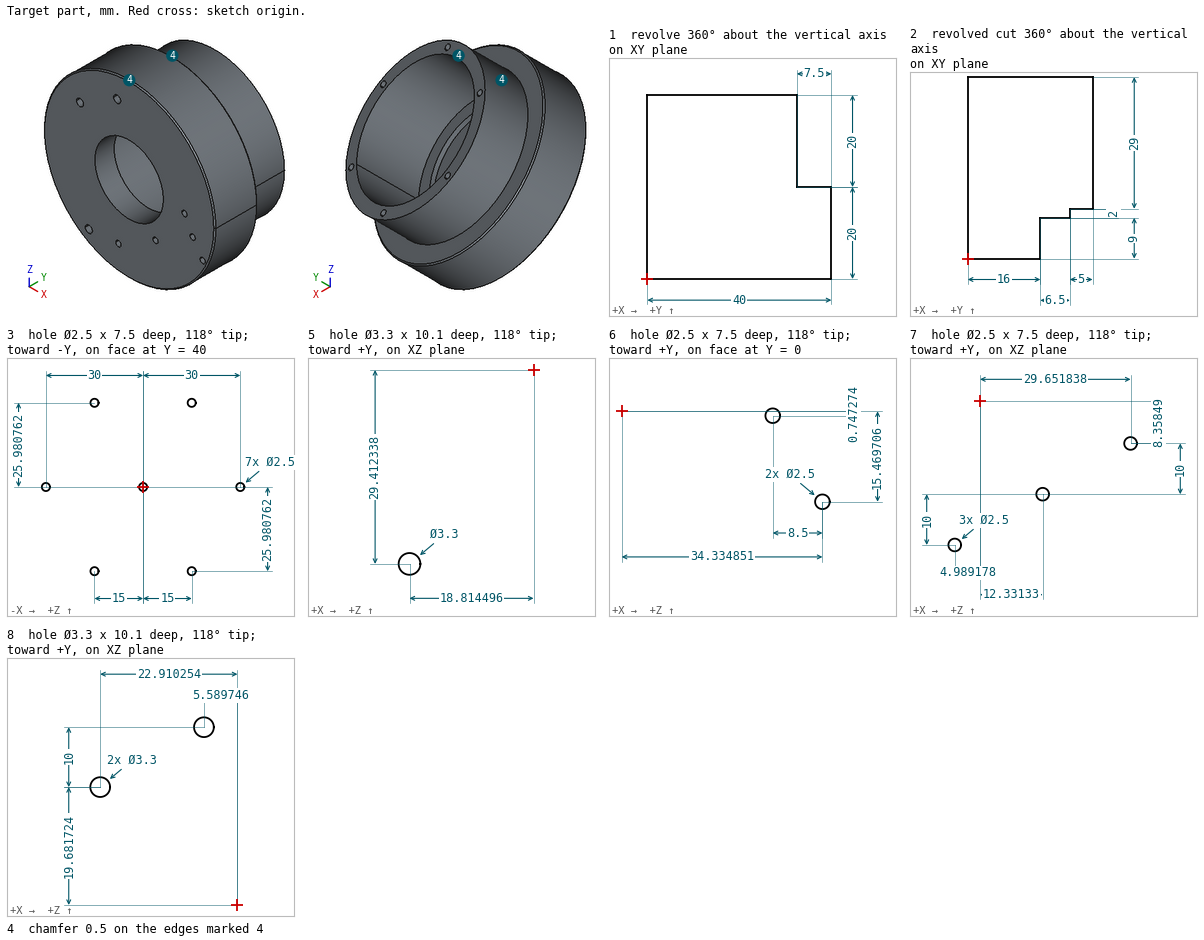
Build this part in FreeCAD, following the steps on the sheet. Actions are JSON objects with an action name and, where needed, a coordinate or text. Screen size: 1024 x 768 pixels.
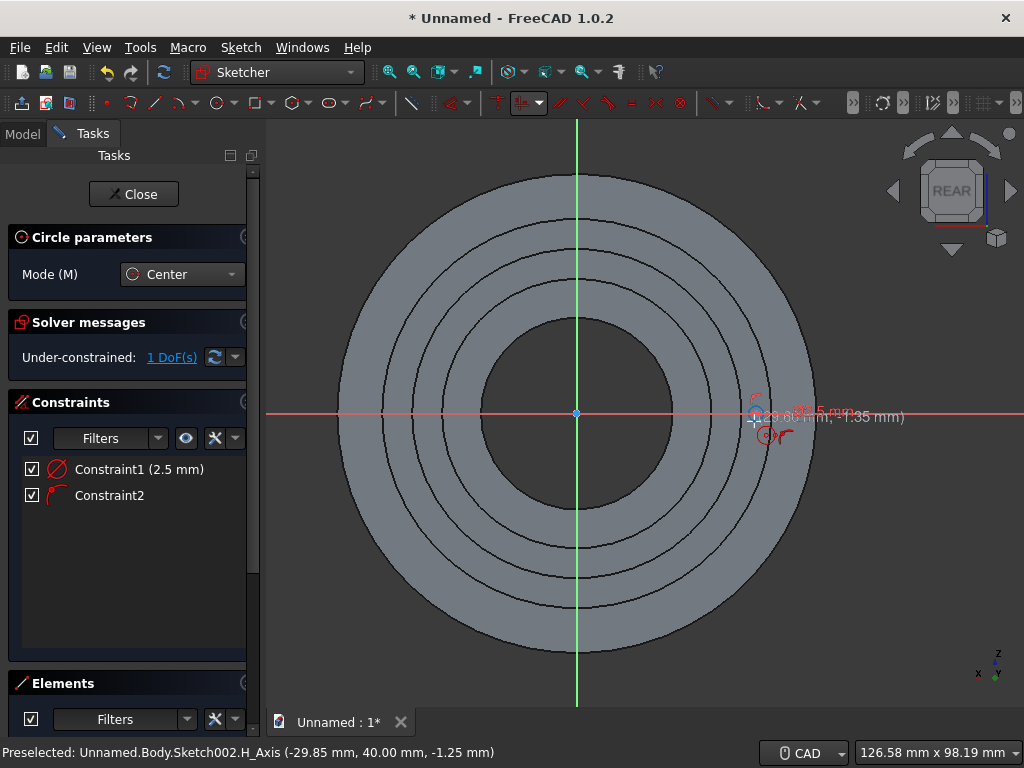
{"action": "scroll", "coordinate": [667, 569], "scroll_direction": "up", "scroll_amount": 6}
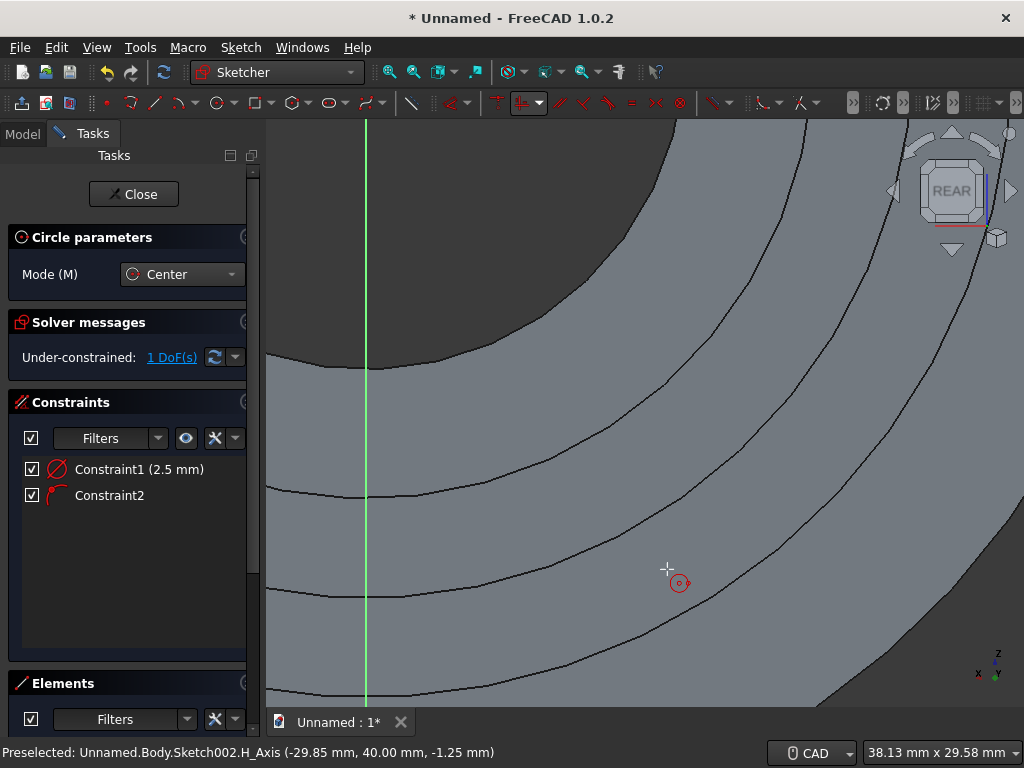
{"action": "scroll", "coordinate": [667, 569], "scroll_direction": "down", "scroll_amount": 6}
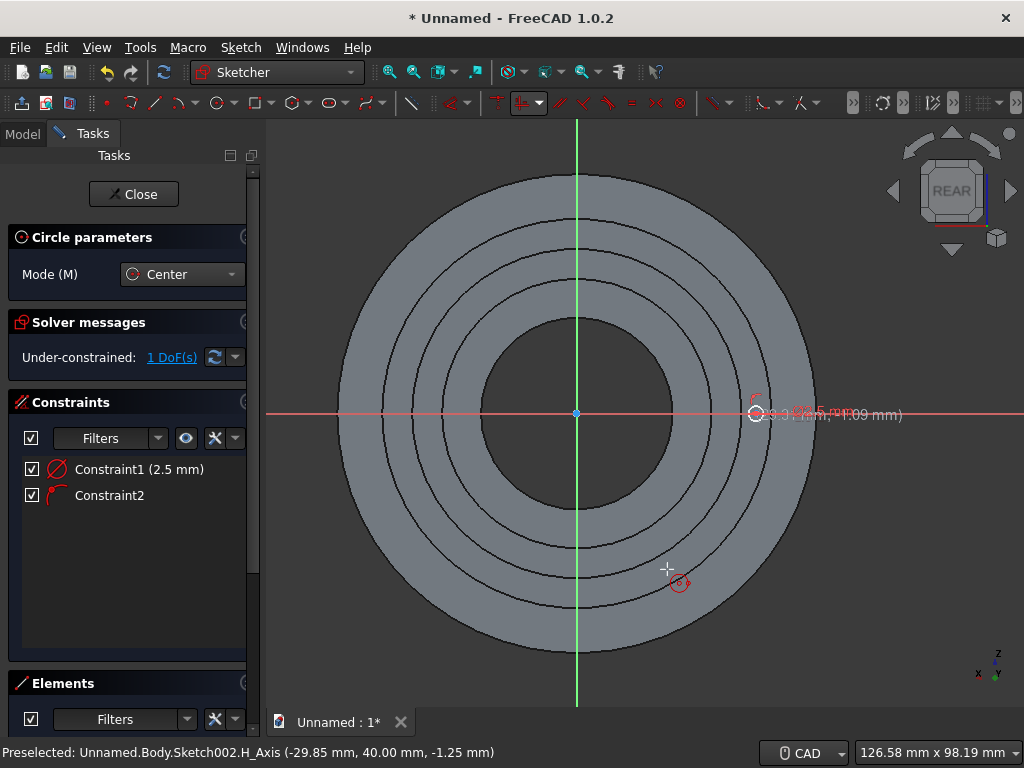
{"action": "left_click", "coordinate": [667, 569]}
{"action": "mouse_move", "coordinate": [672, 564]}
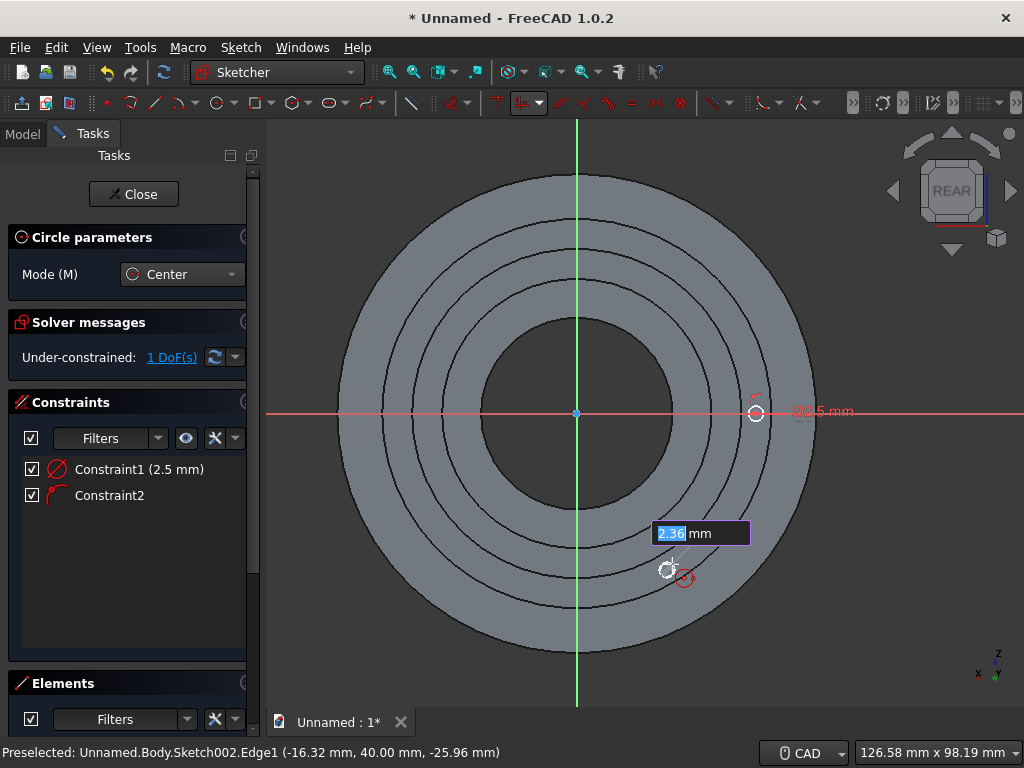
{"action": "type", "text": "2.5"}
{"action": "key", "text": "Return"}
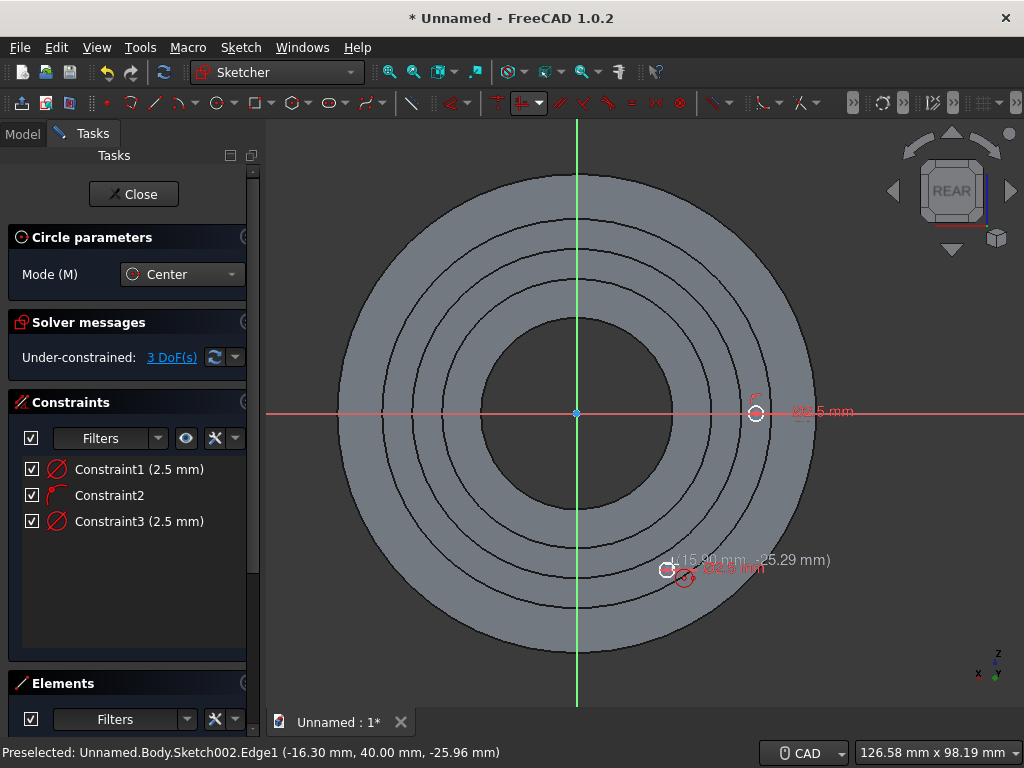
{"action": "scroll", "coordinate": [487, 569], "scroll_direction": "up", "scroll_amount": 6}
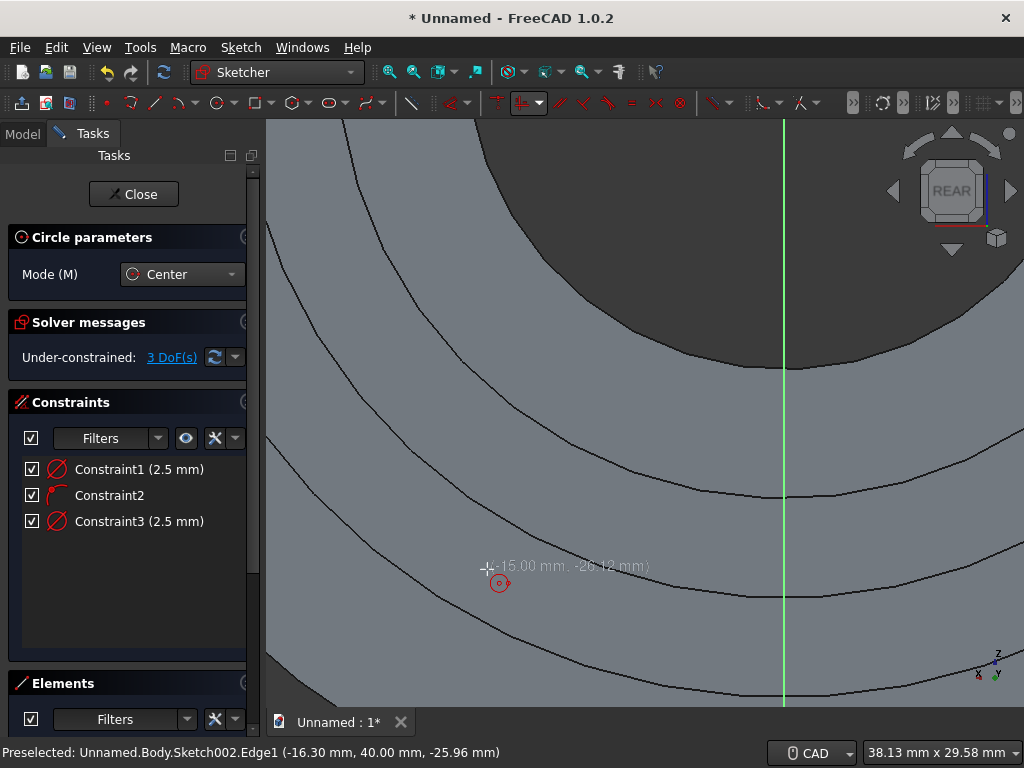
{"action": "scroll", "coordinate": [487, 569], "scroll_direction": "down", "scroll_amount": 6}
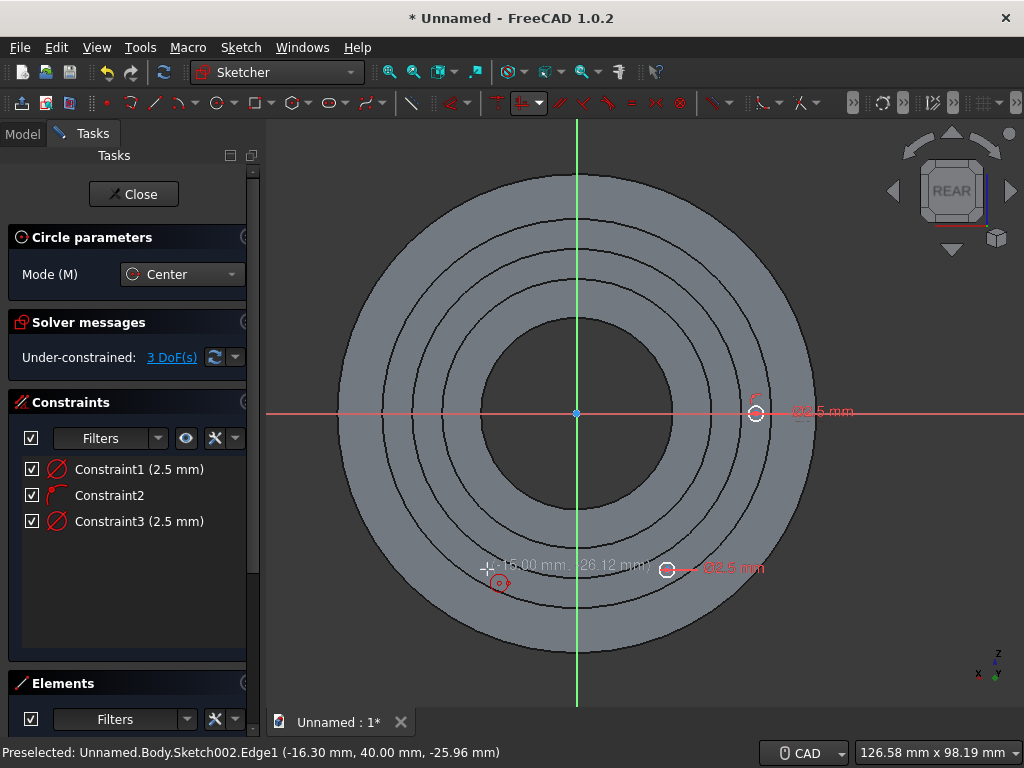
{"action": "left_click", "coordinate": [487, 569]}
{"action": "mouse_move", "coordinate": [492, 564]}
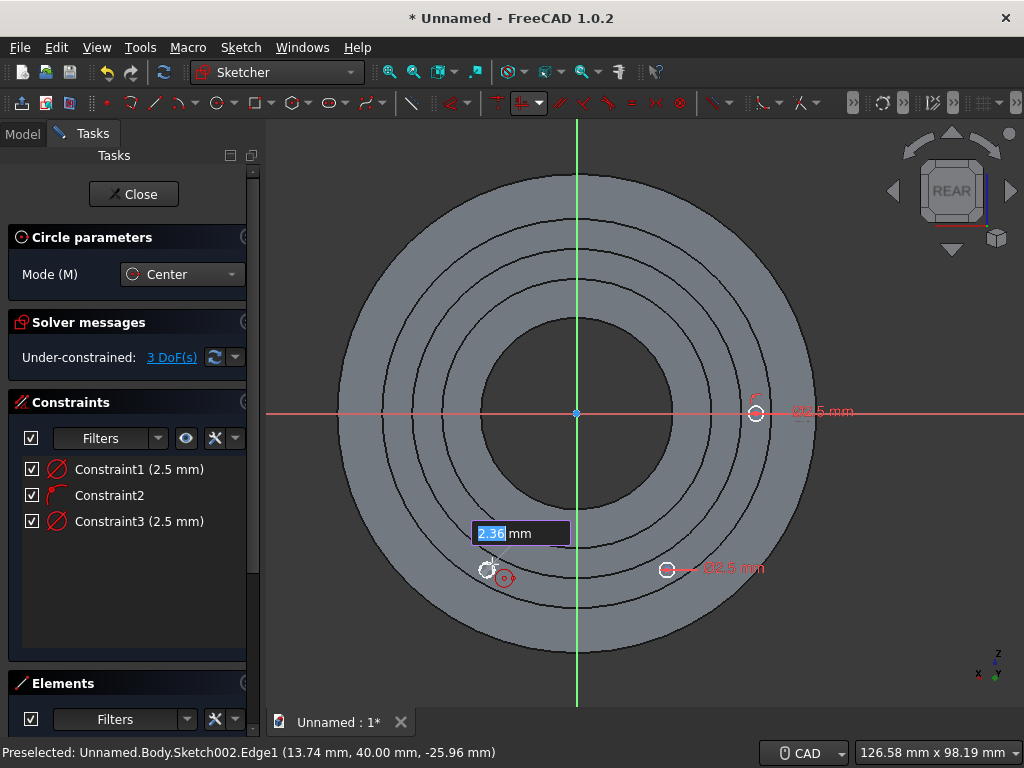
{"action": "type", "text": "2.5"}
{"action": "key", "text": "Return"}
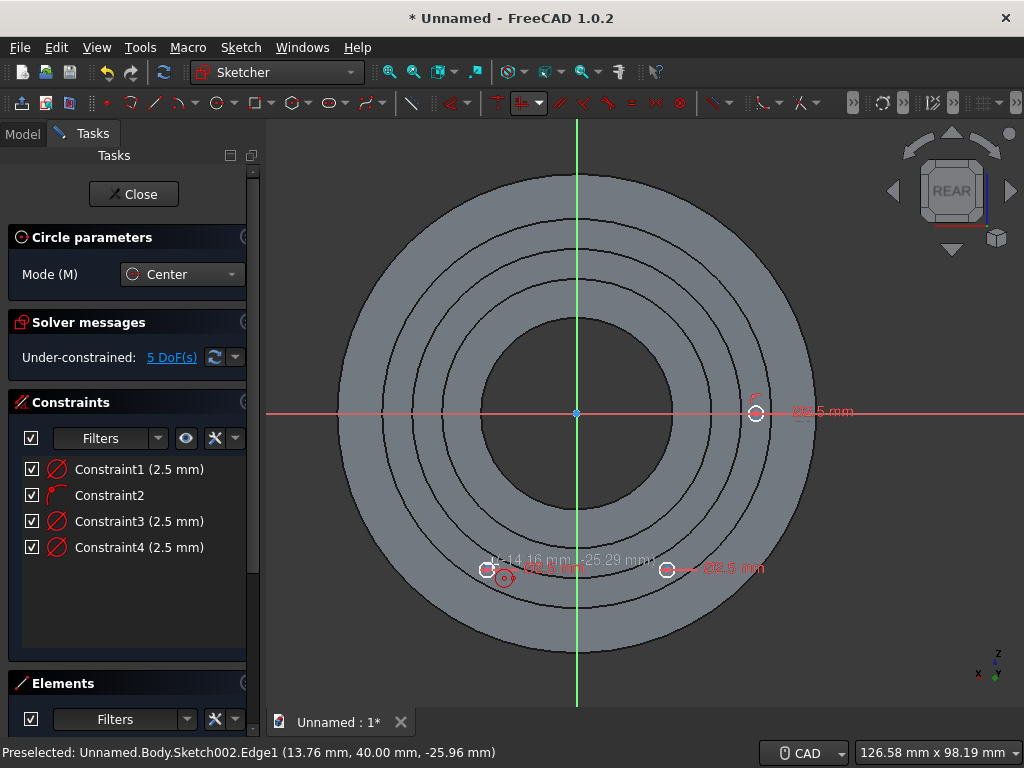
{"action": "scroll", "coordinate": [397, 414], "scroll_direction": "up", "scroll_amount": 6}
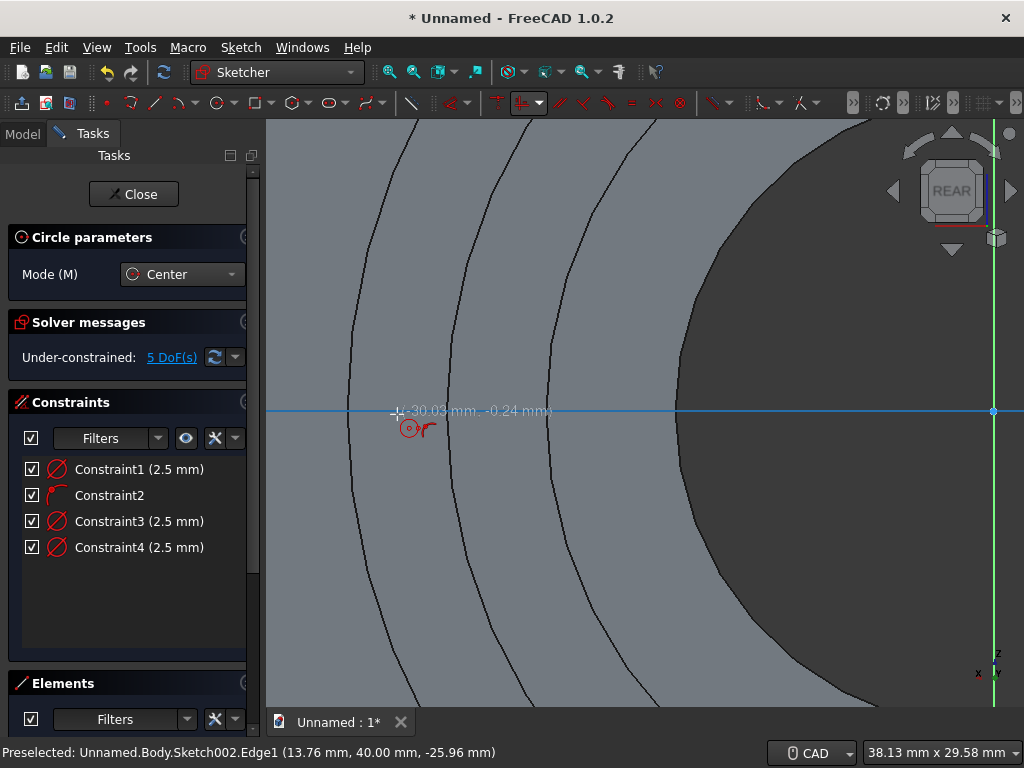
{"action": "scroll", "coordinate": [397, 414], "scroll_direction": "down", "scroll_amount": 6}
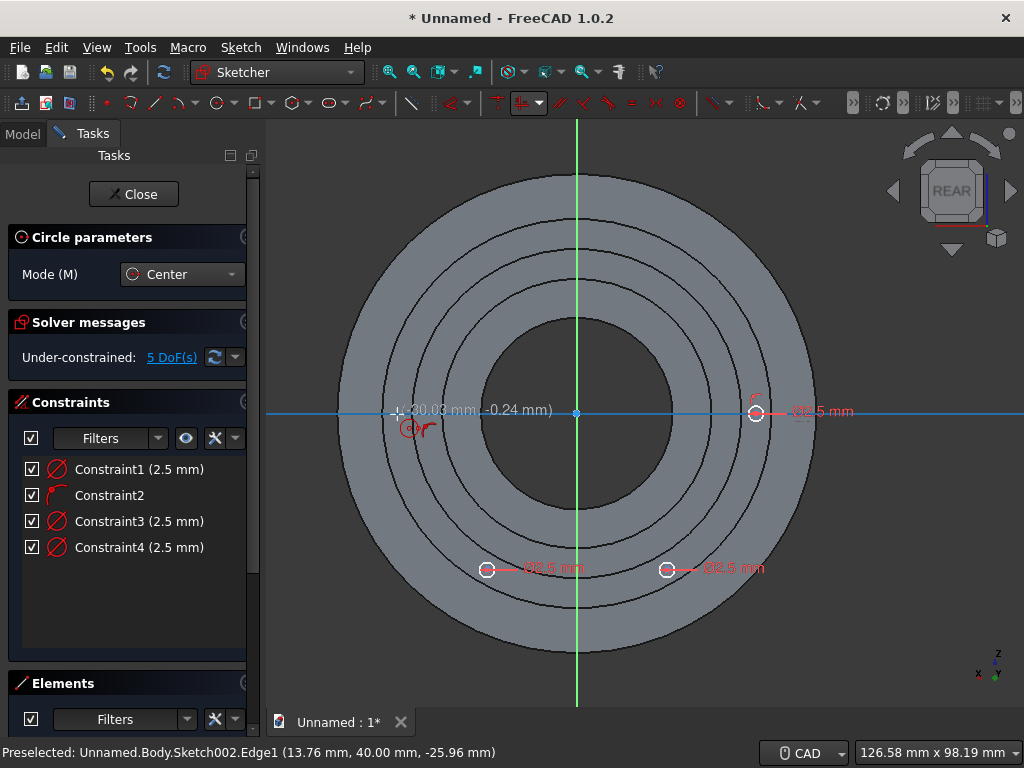
{"action": "left_click", "coordinate": [397, 414]}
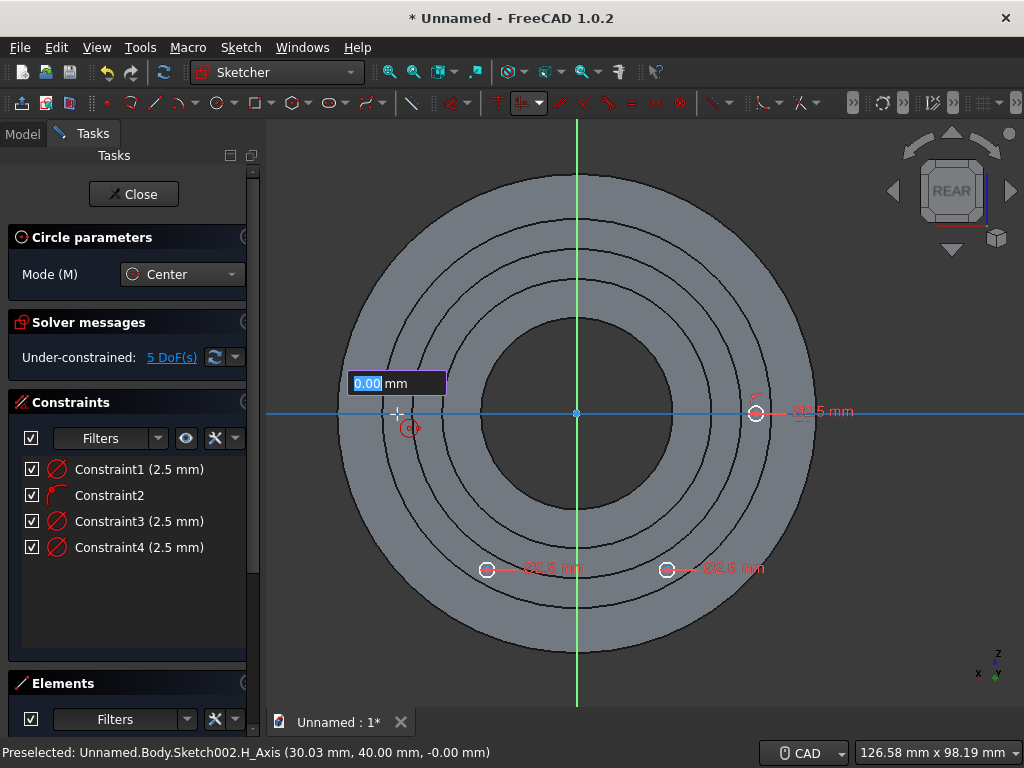
{"action": "scroll", "coordinate": [395, 421], "scroll_direction": "up", "scroll_amount": 5}
{"action": "mouse_move", "coordinate": [394, 419]}